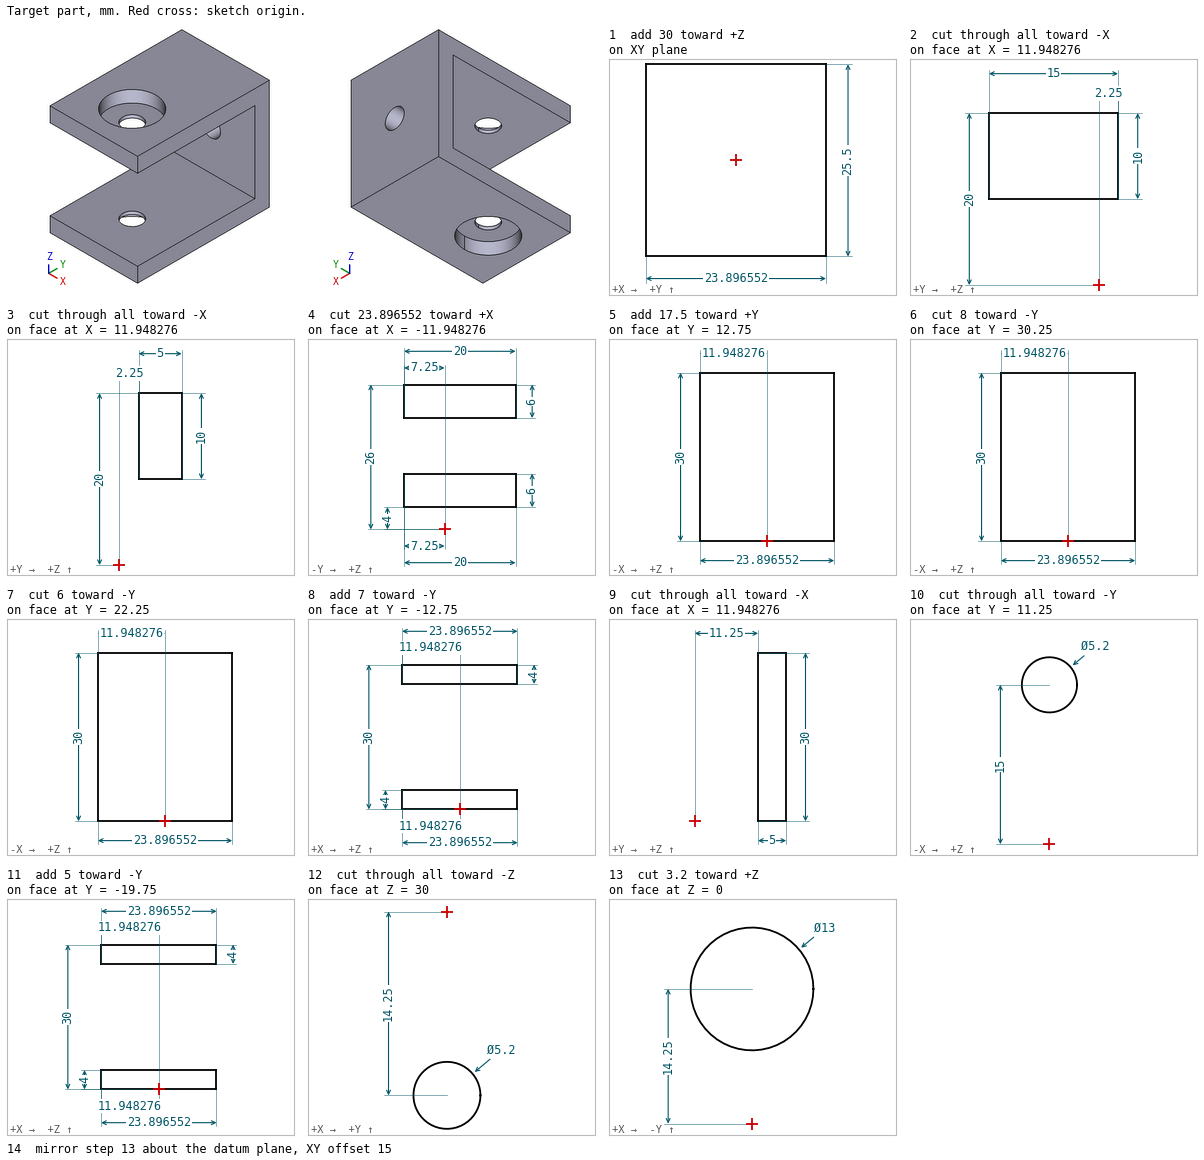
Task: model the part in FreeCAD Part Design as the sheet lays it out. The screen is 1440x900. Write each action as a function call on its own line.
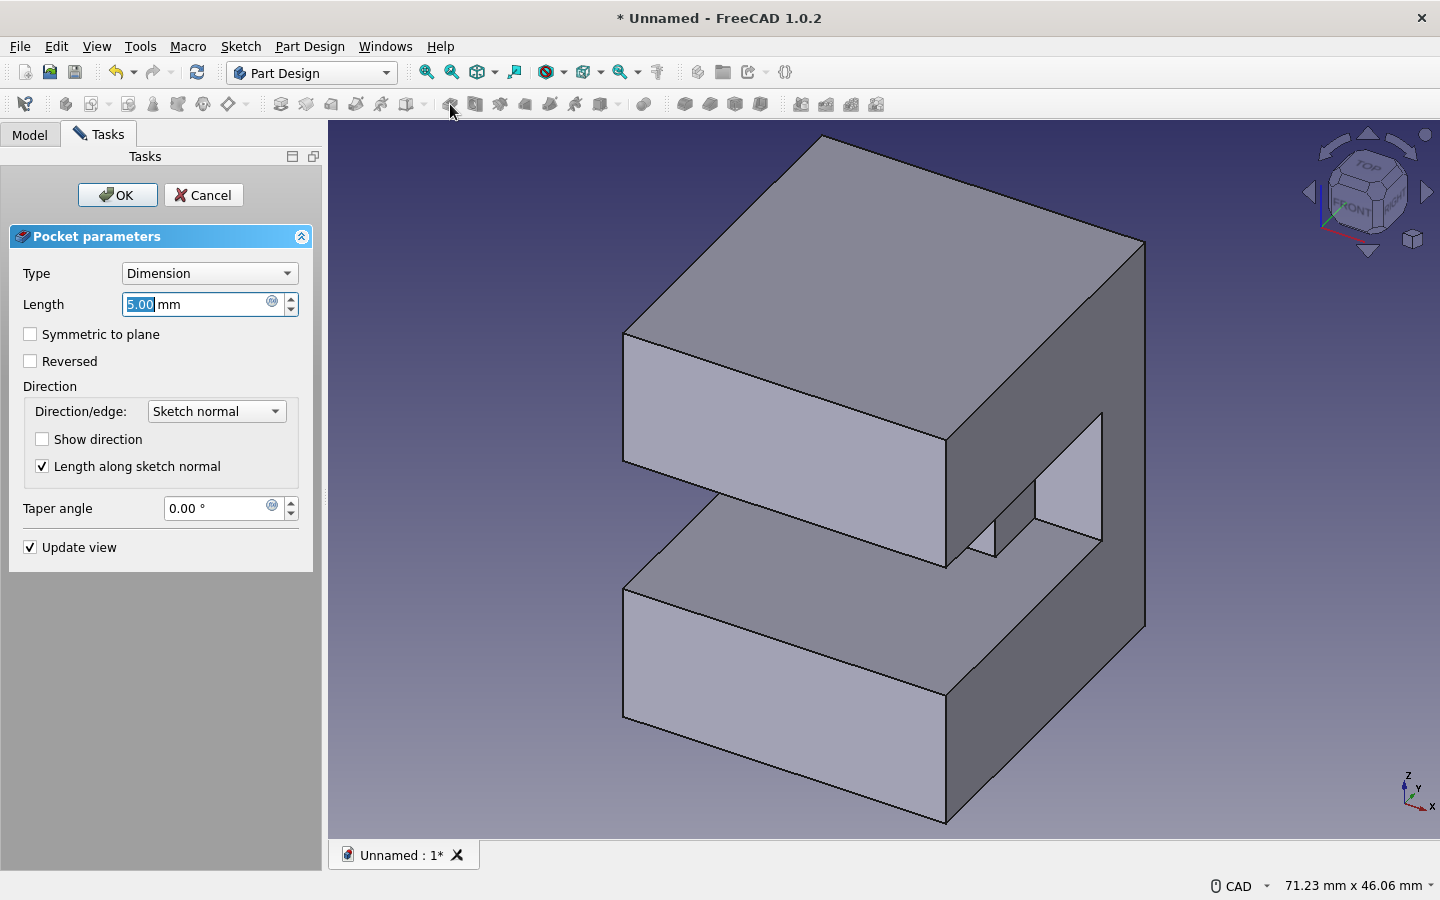
click(210, 274)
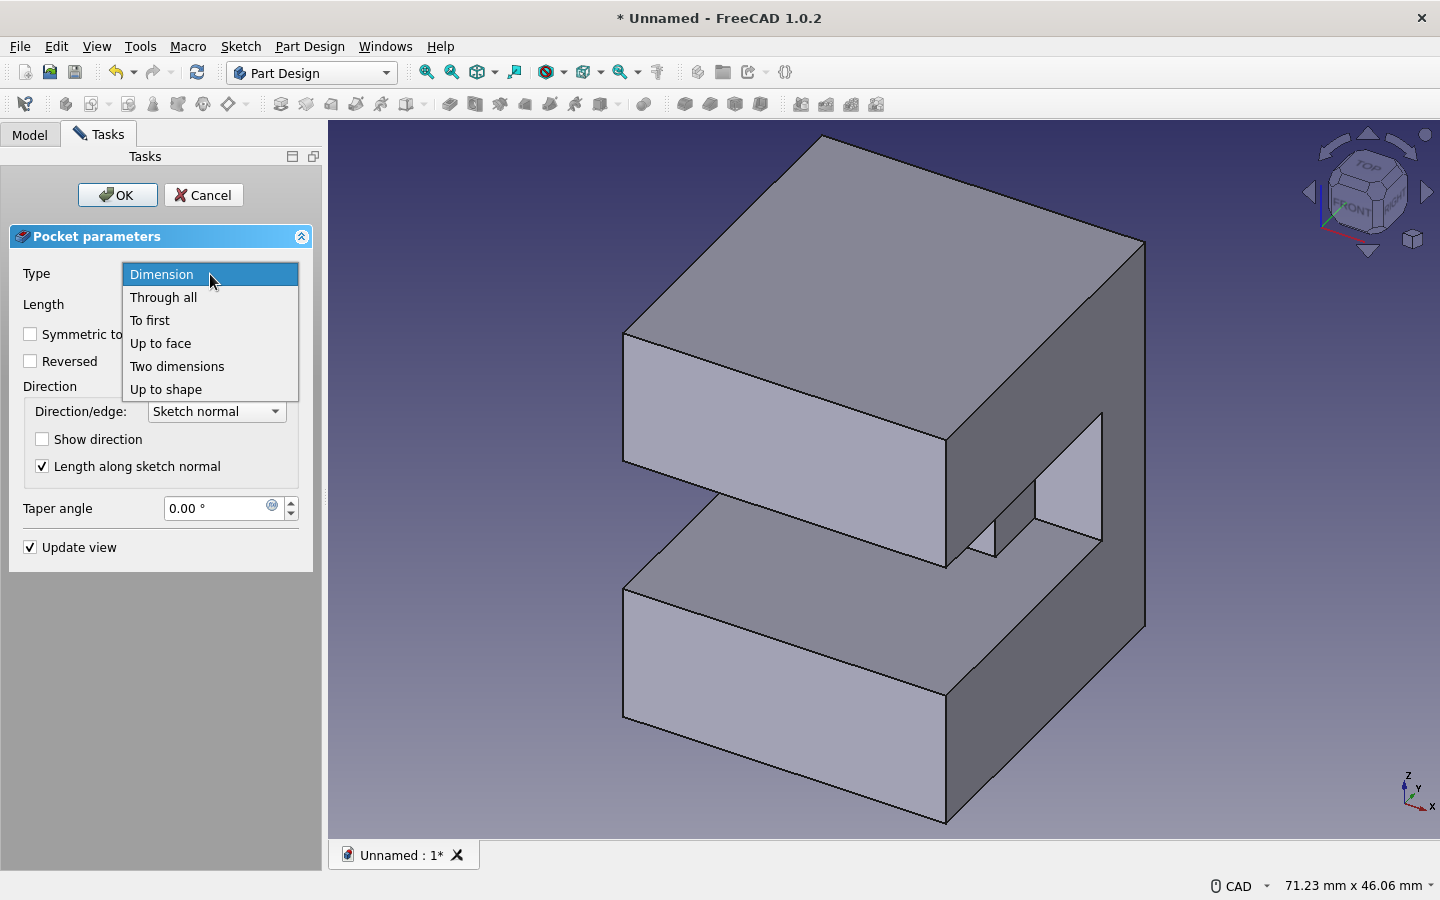
click(208, 298)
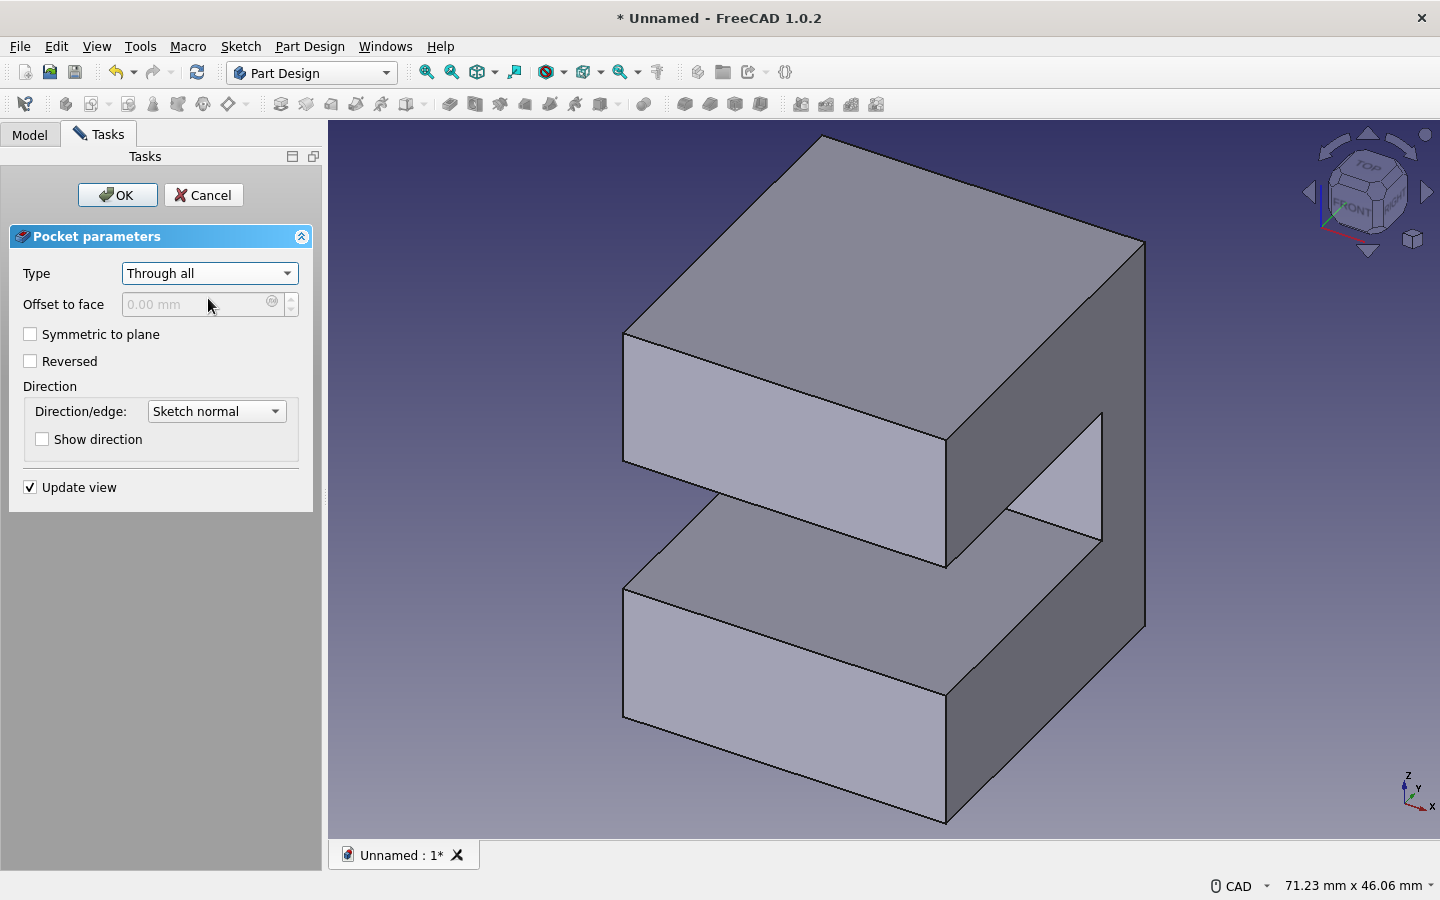
click(118, 195)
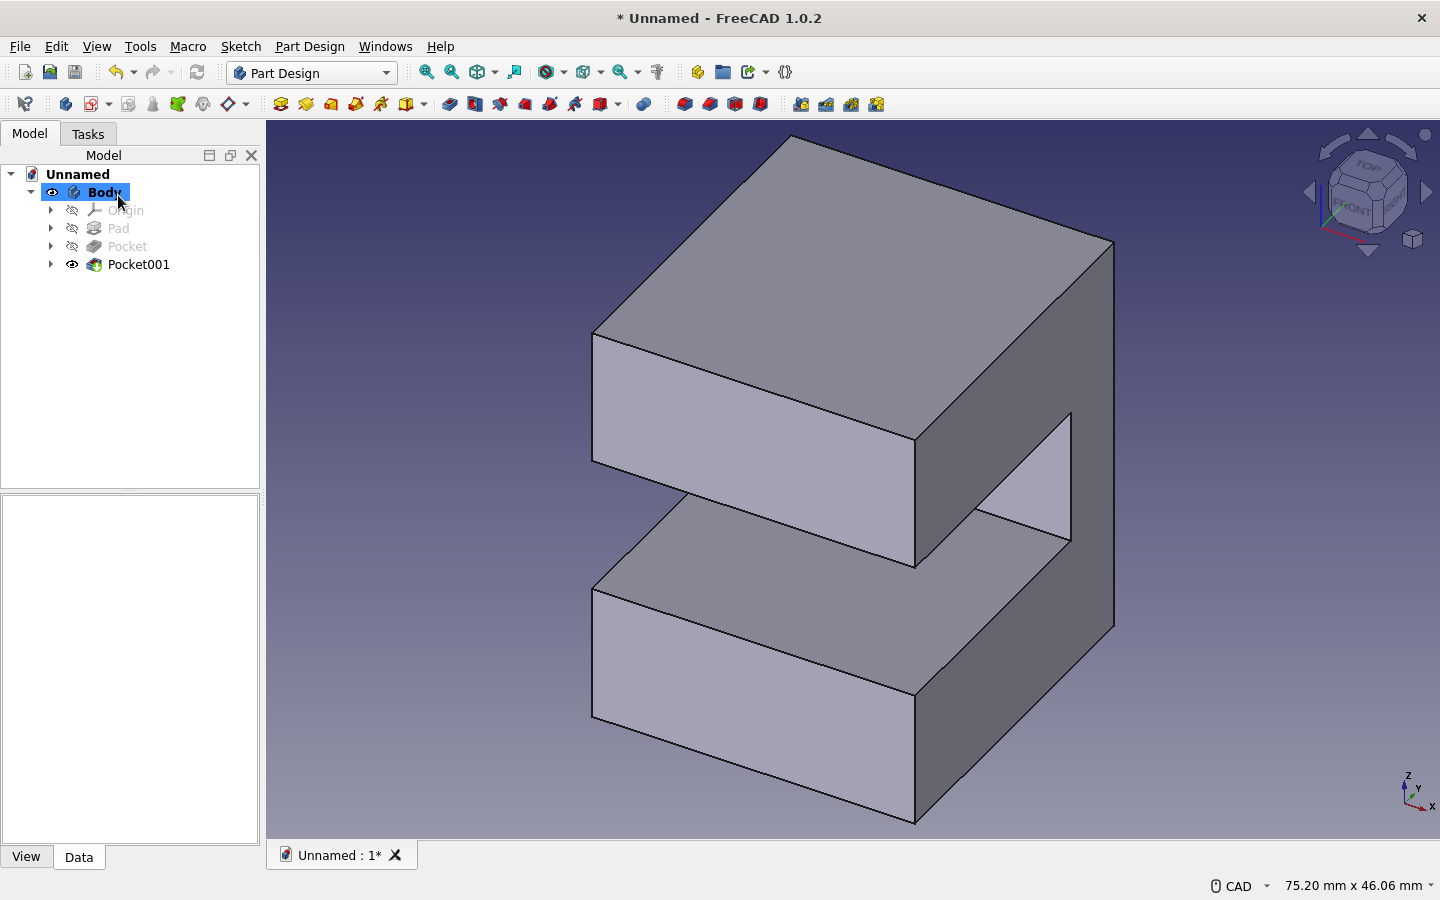
key(6)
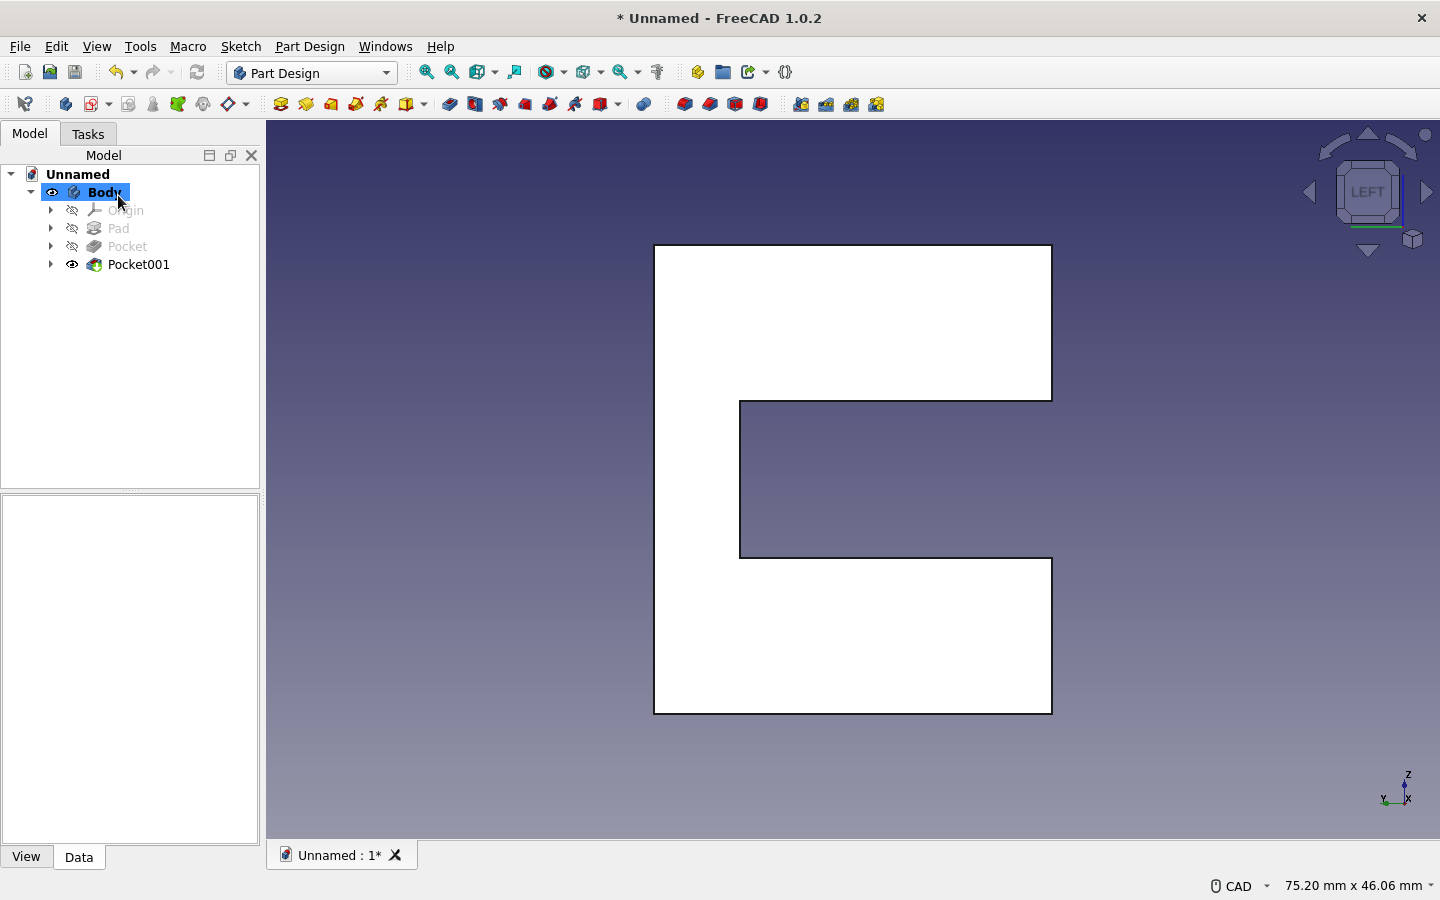
click(739, 612)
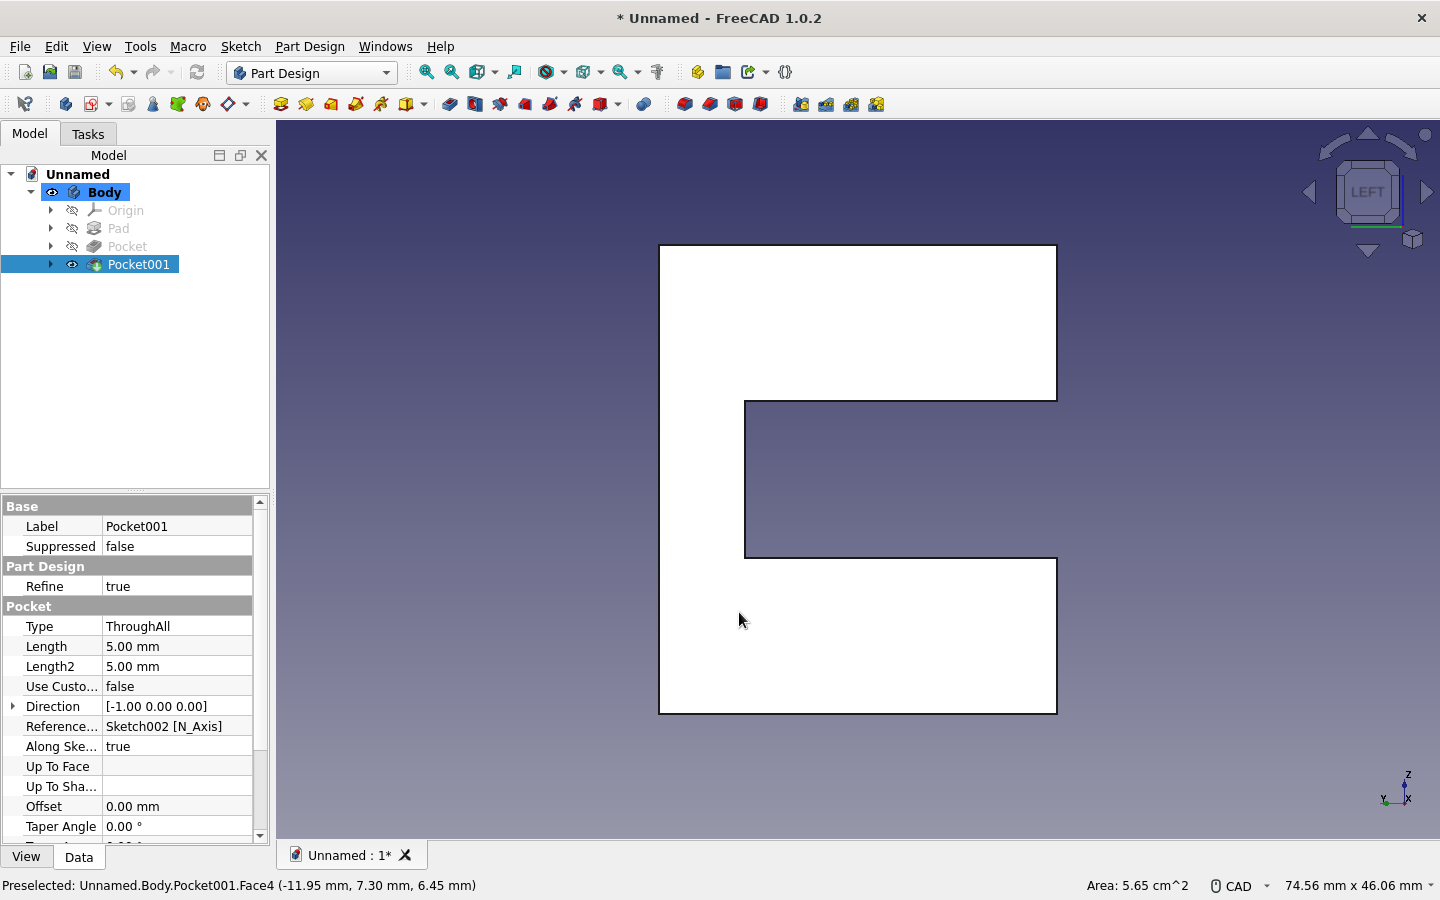
click(90, 104)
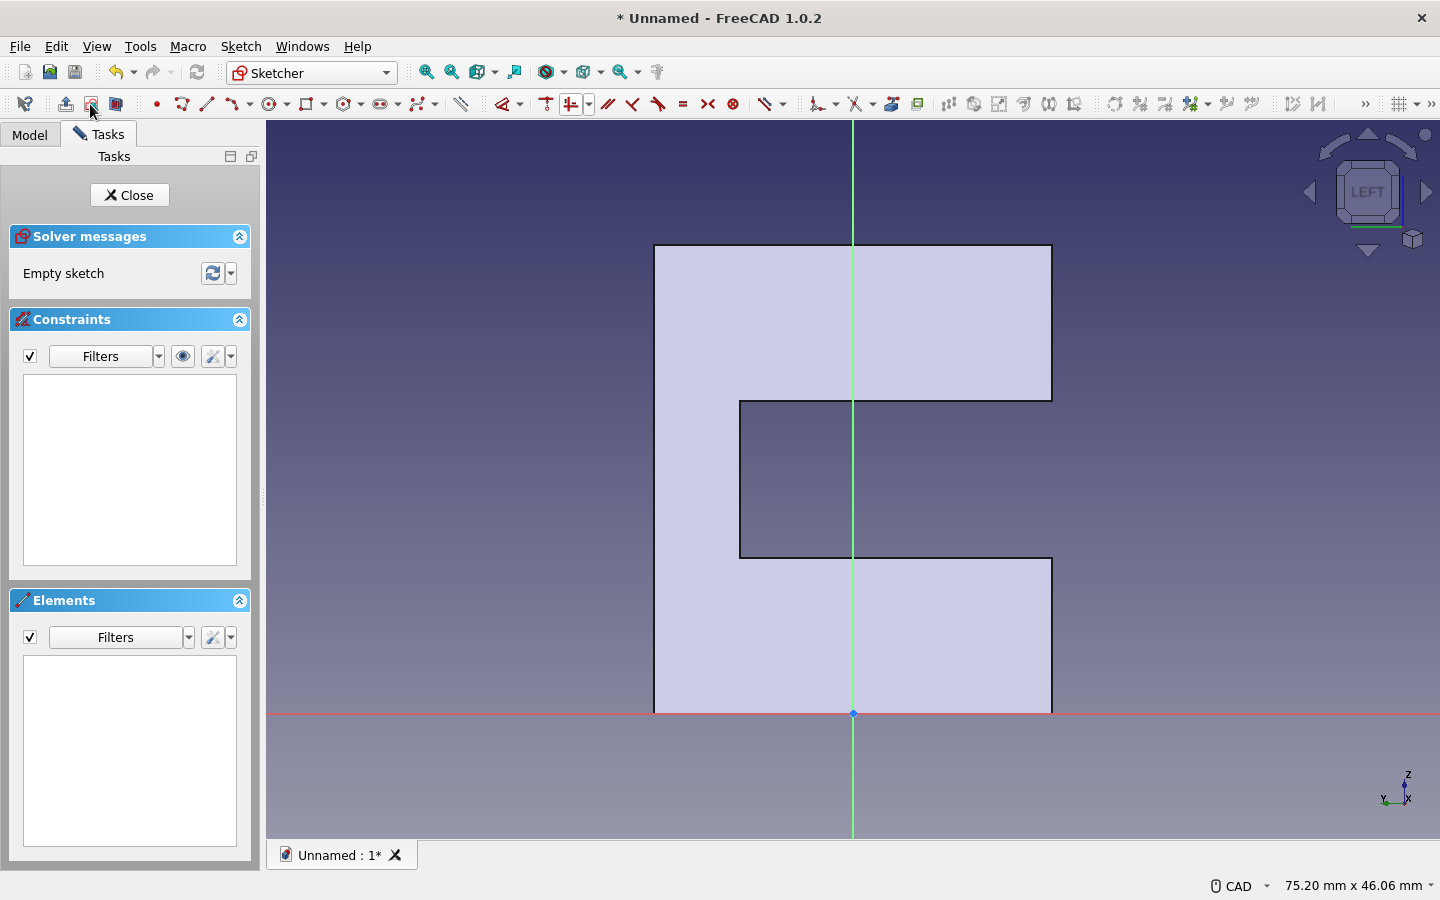
key(g)
key(r)